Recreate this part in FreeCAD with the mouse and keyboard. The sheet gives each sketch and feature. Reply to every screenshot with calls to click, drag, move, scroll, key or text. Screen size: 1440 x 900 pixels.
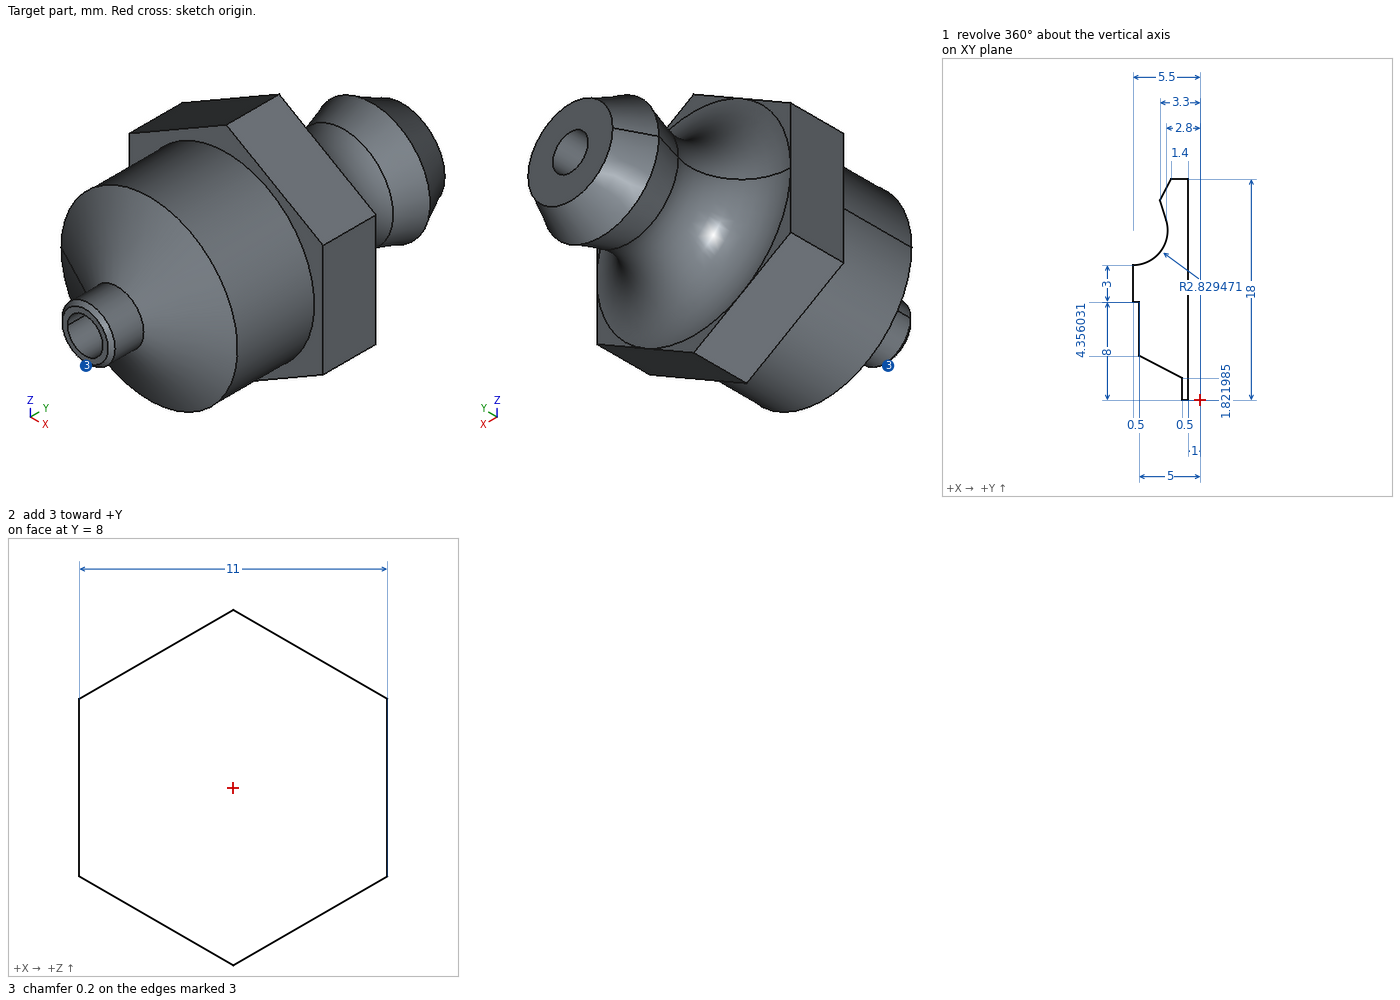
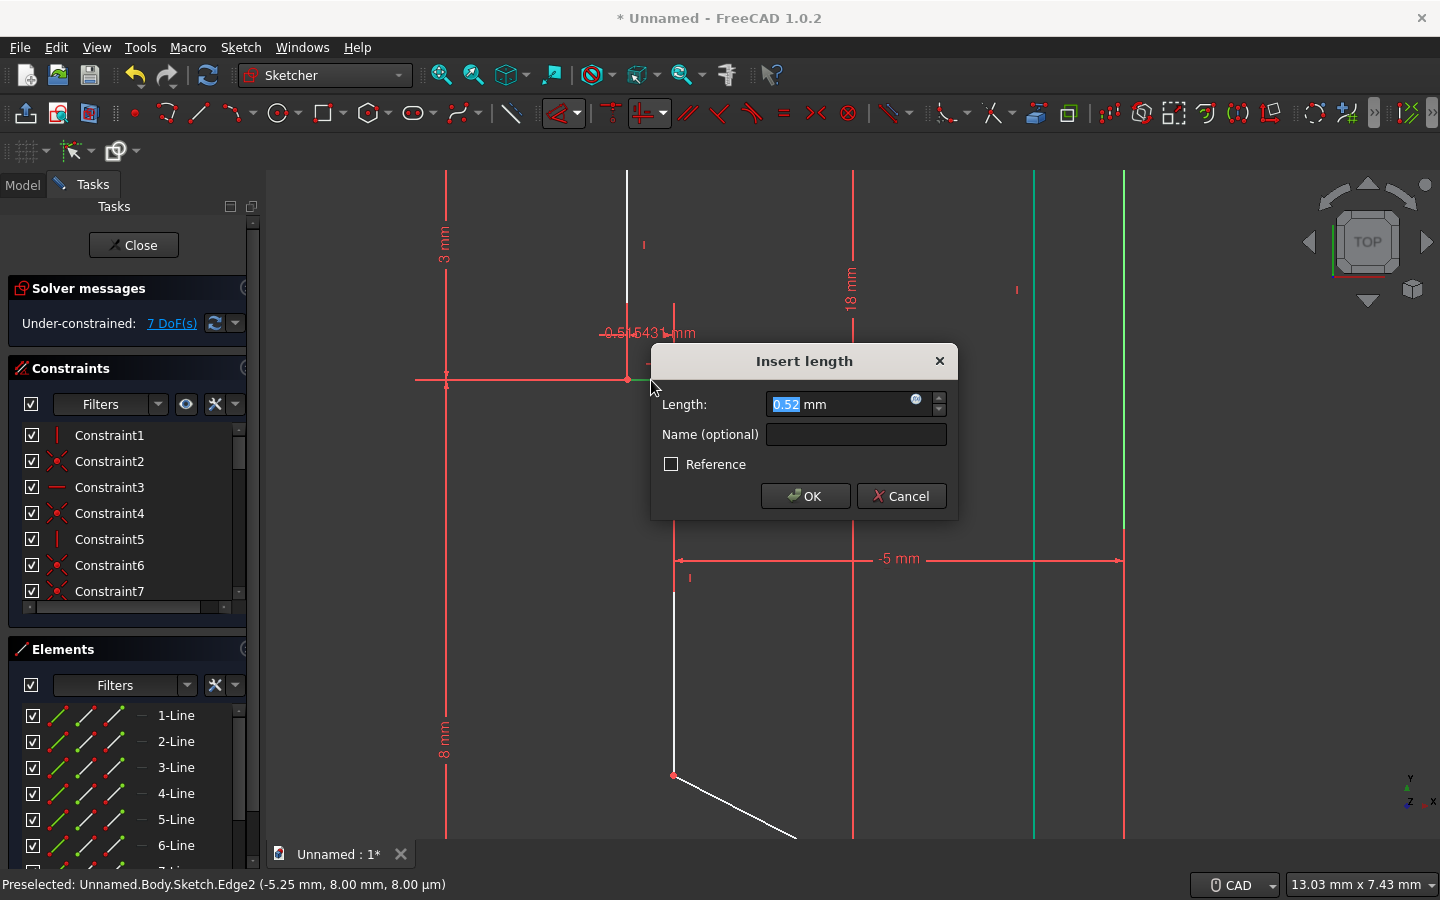
text(0.5)
key(Return)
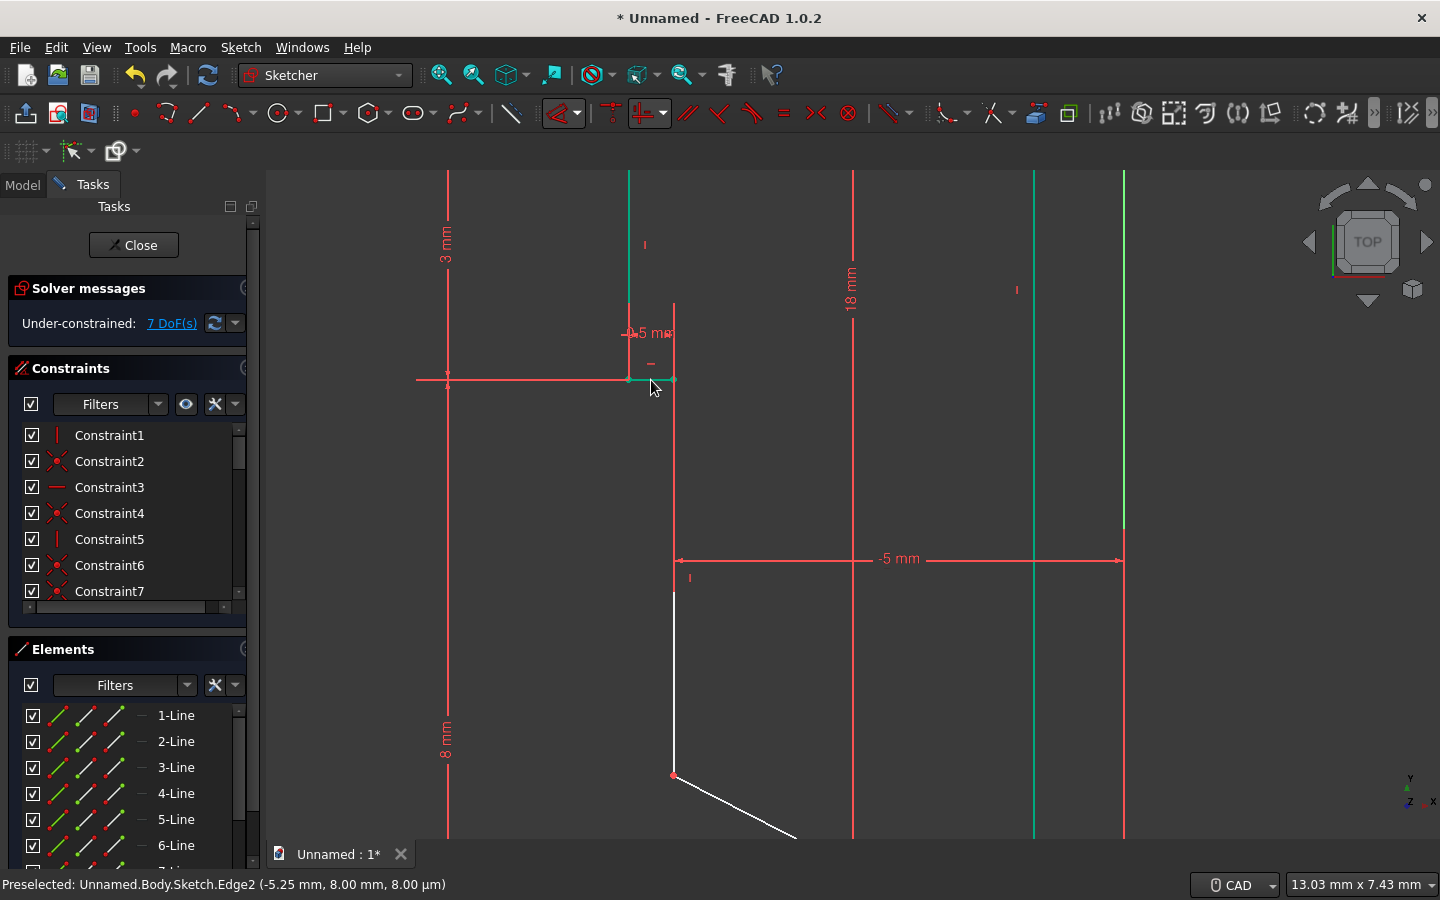
scroll(754, 575, down, 7)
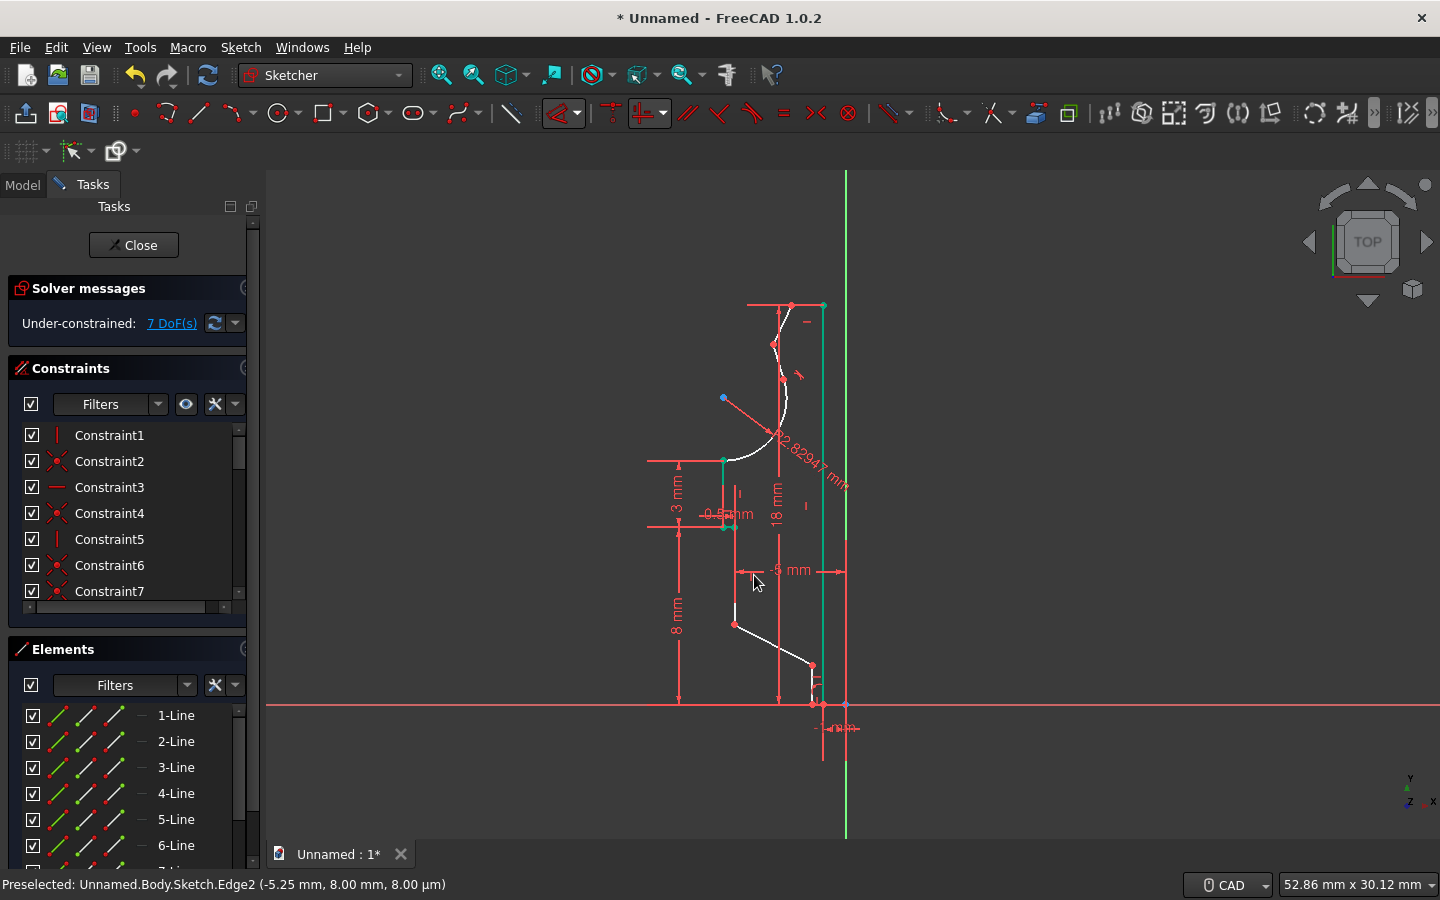
scroll(816, 705, up, 8)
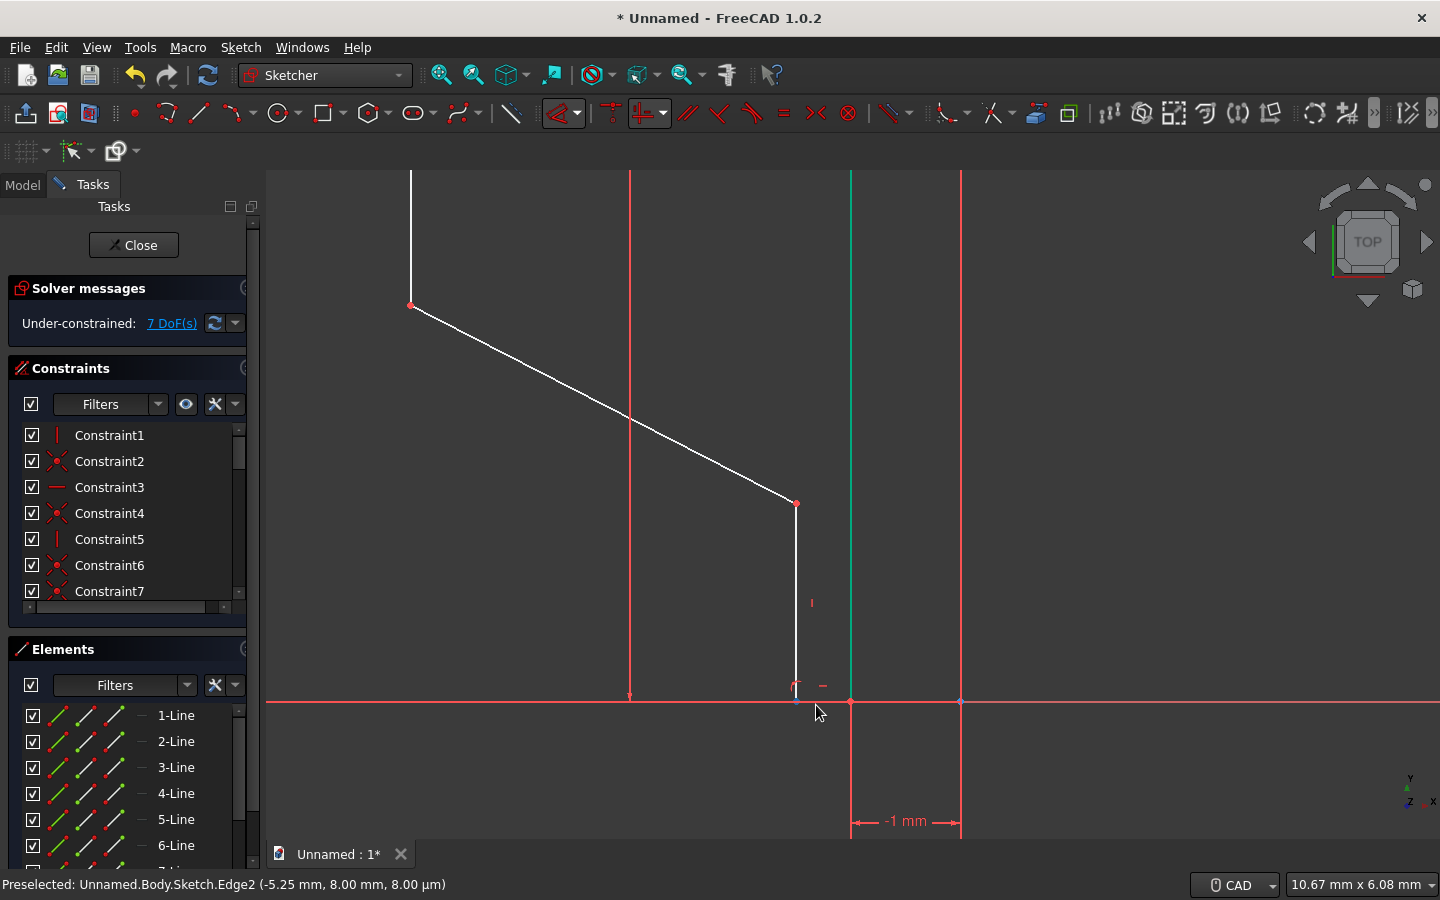
click(812, 702)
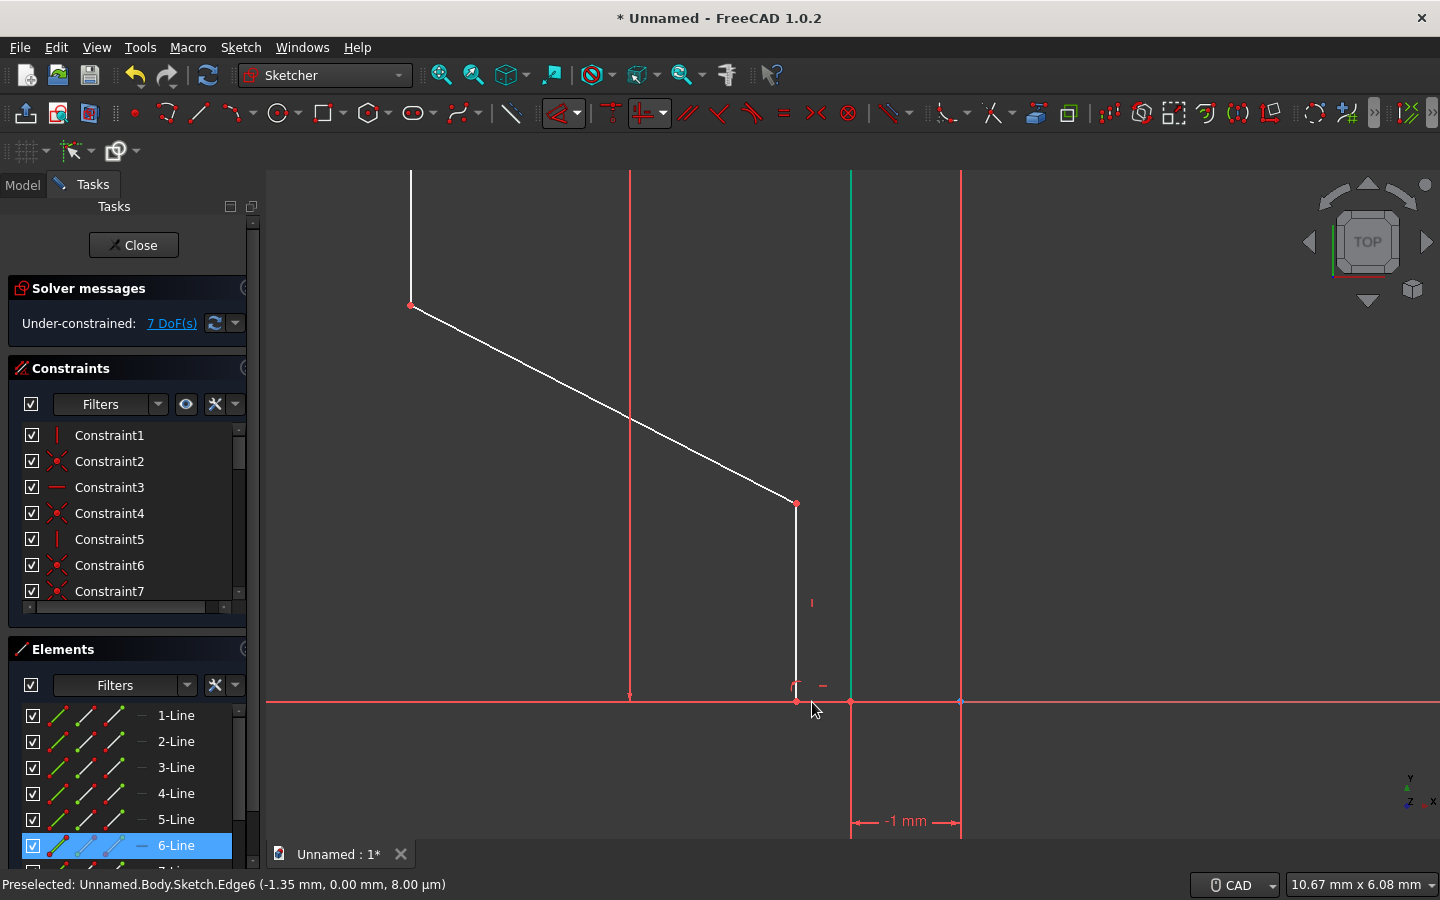
click(580, 114)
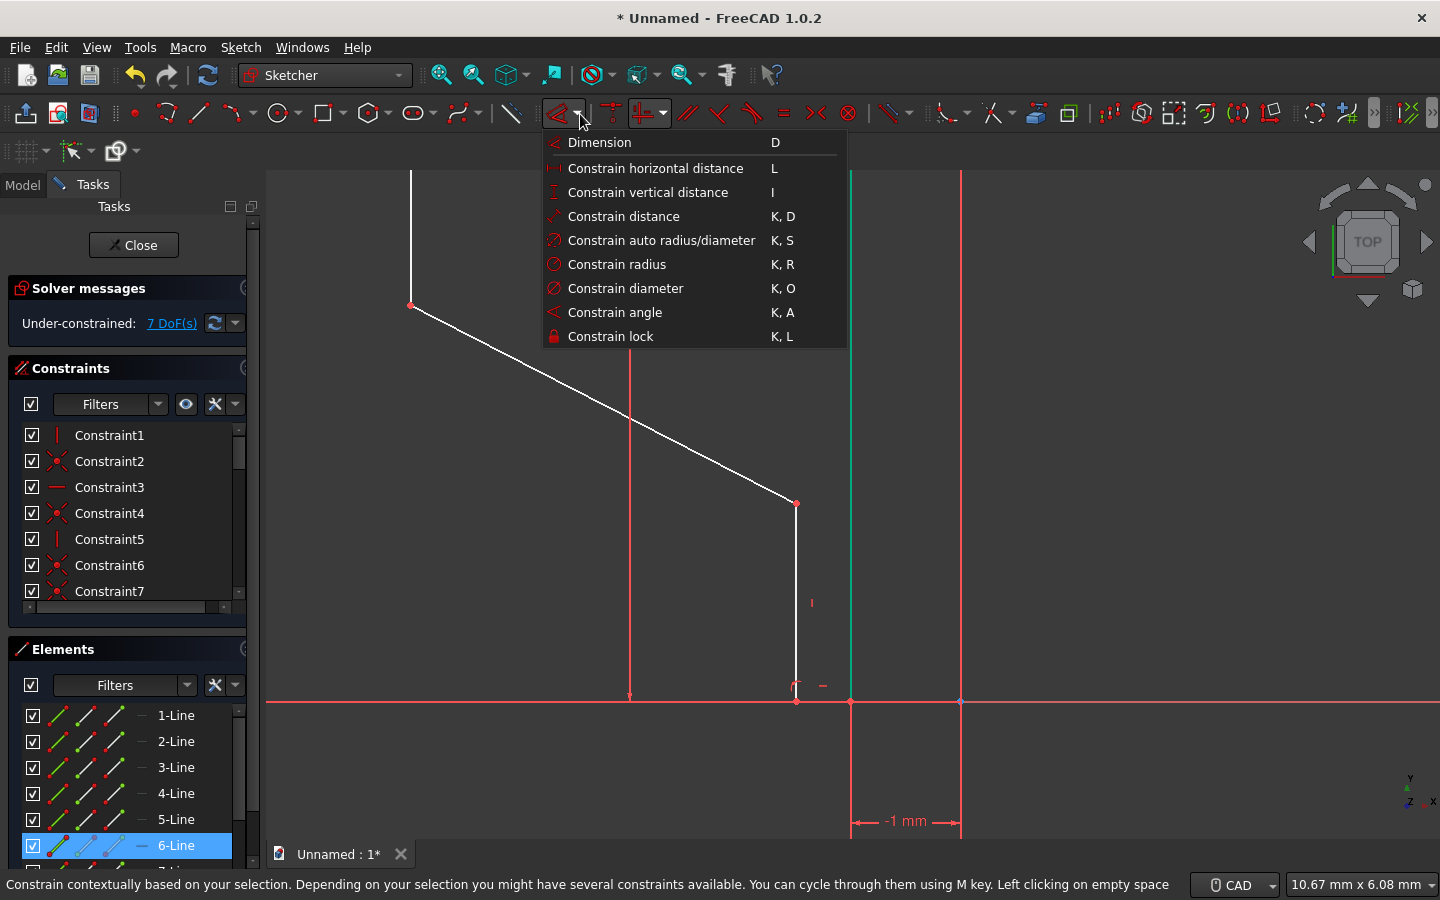
click(695, 168)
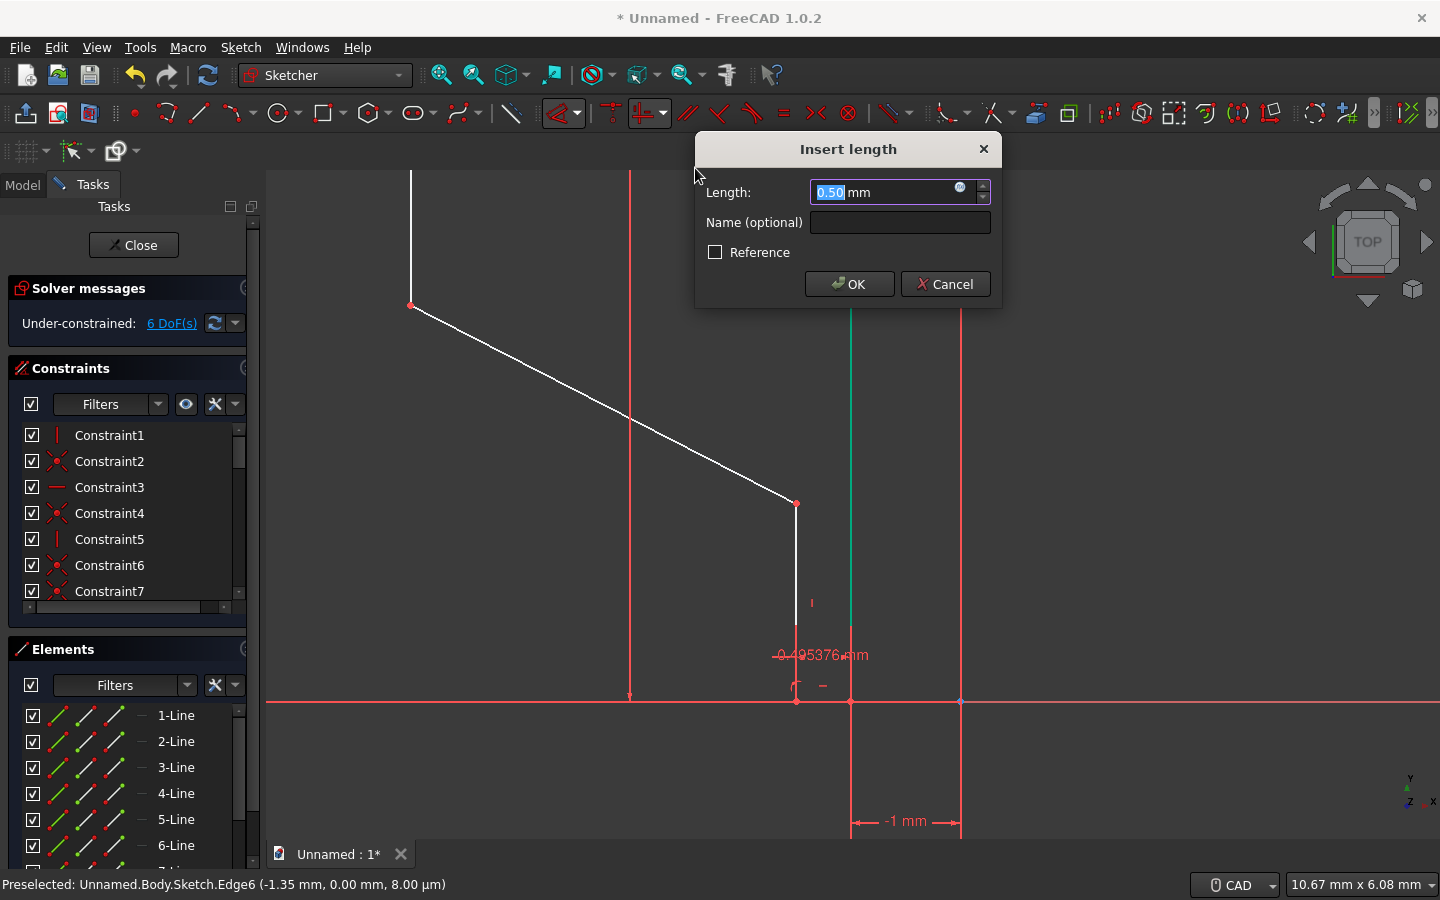
text(0.5)
key(Return)